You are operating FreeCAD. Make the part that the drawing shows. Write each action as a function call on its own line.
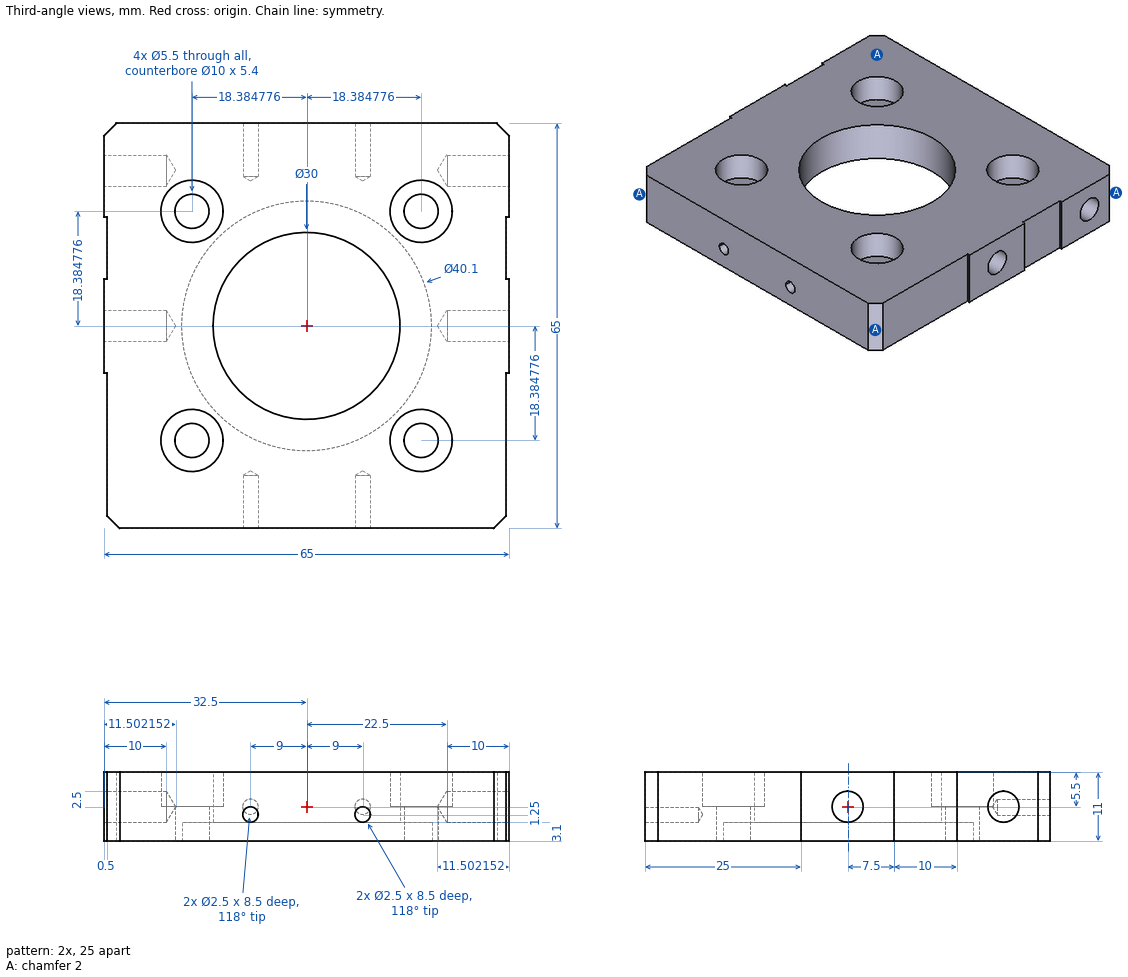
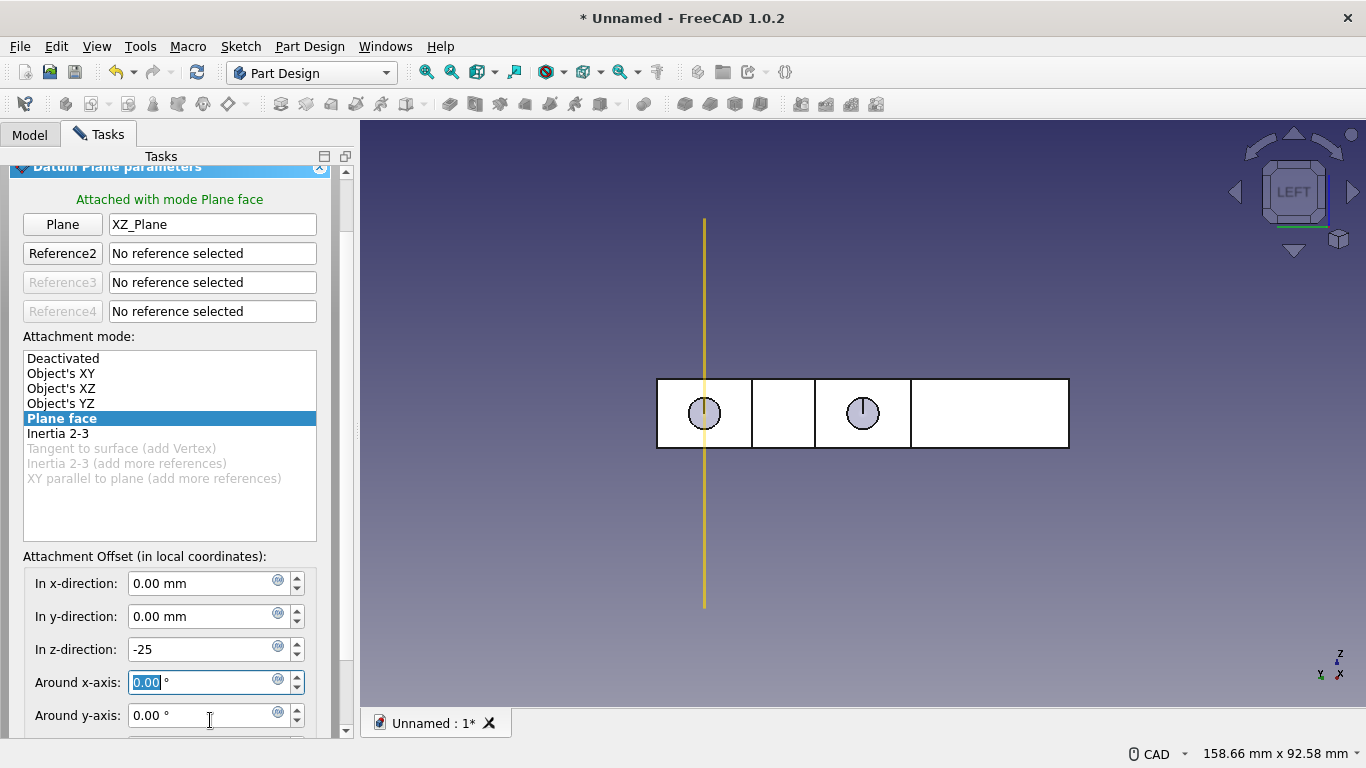
scroll(346, 452, up, 2)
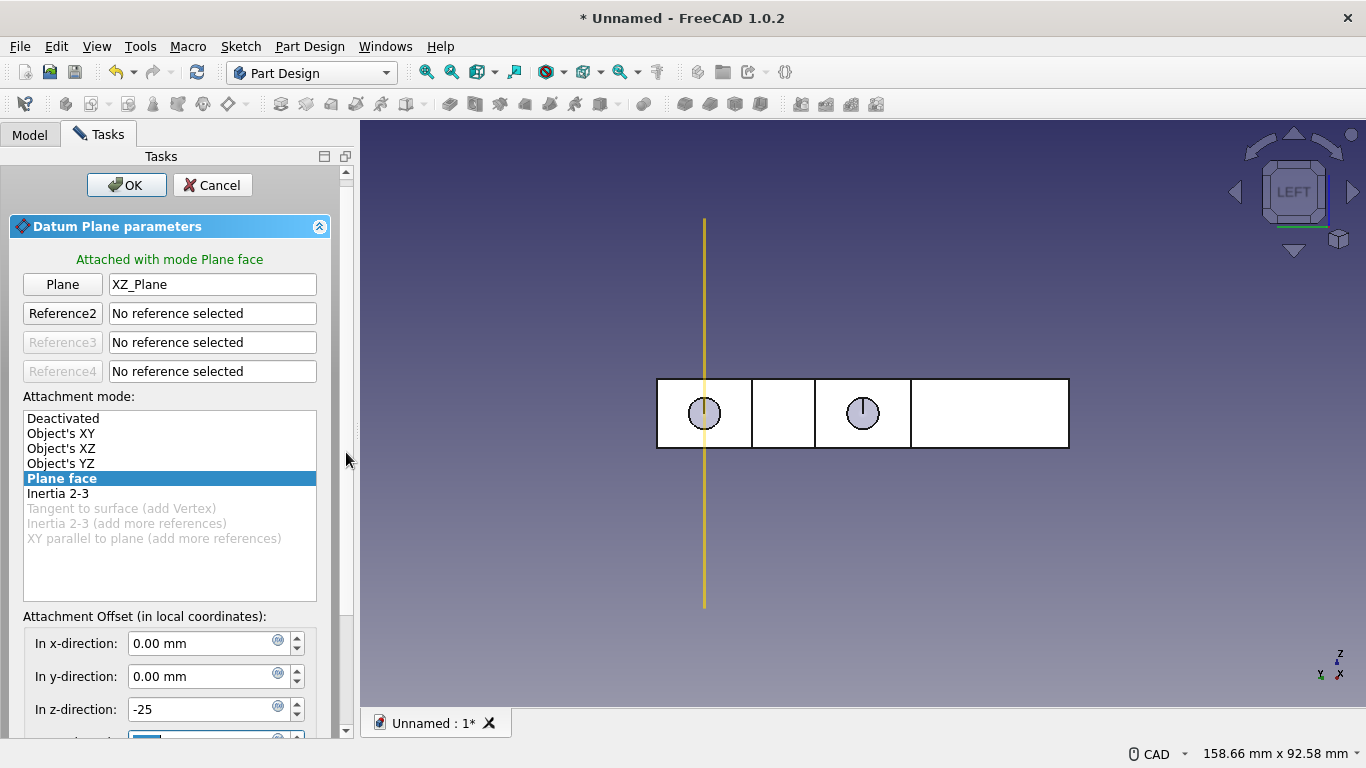
click(127, 195)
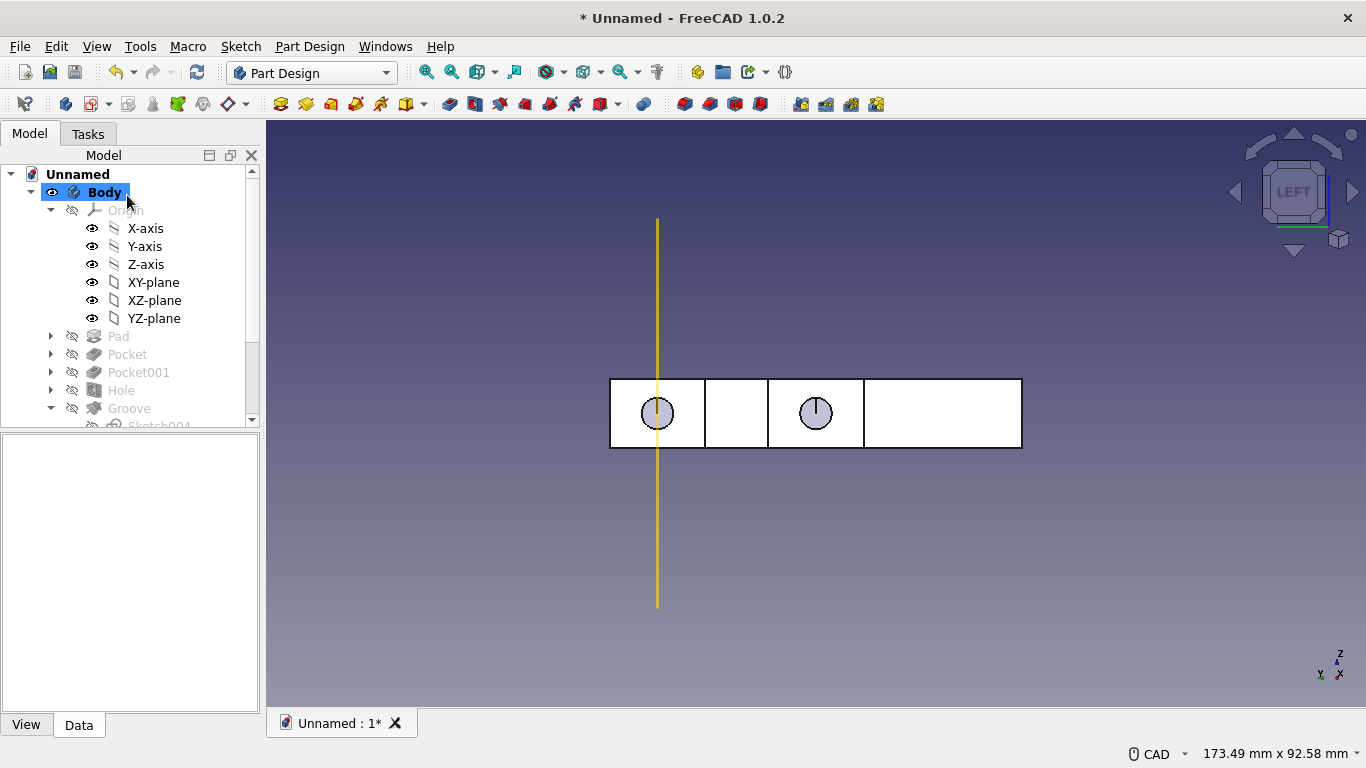
scroll(101, 296, down, 3)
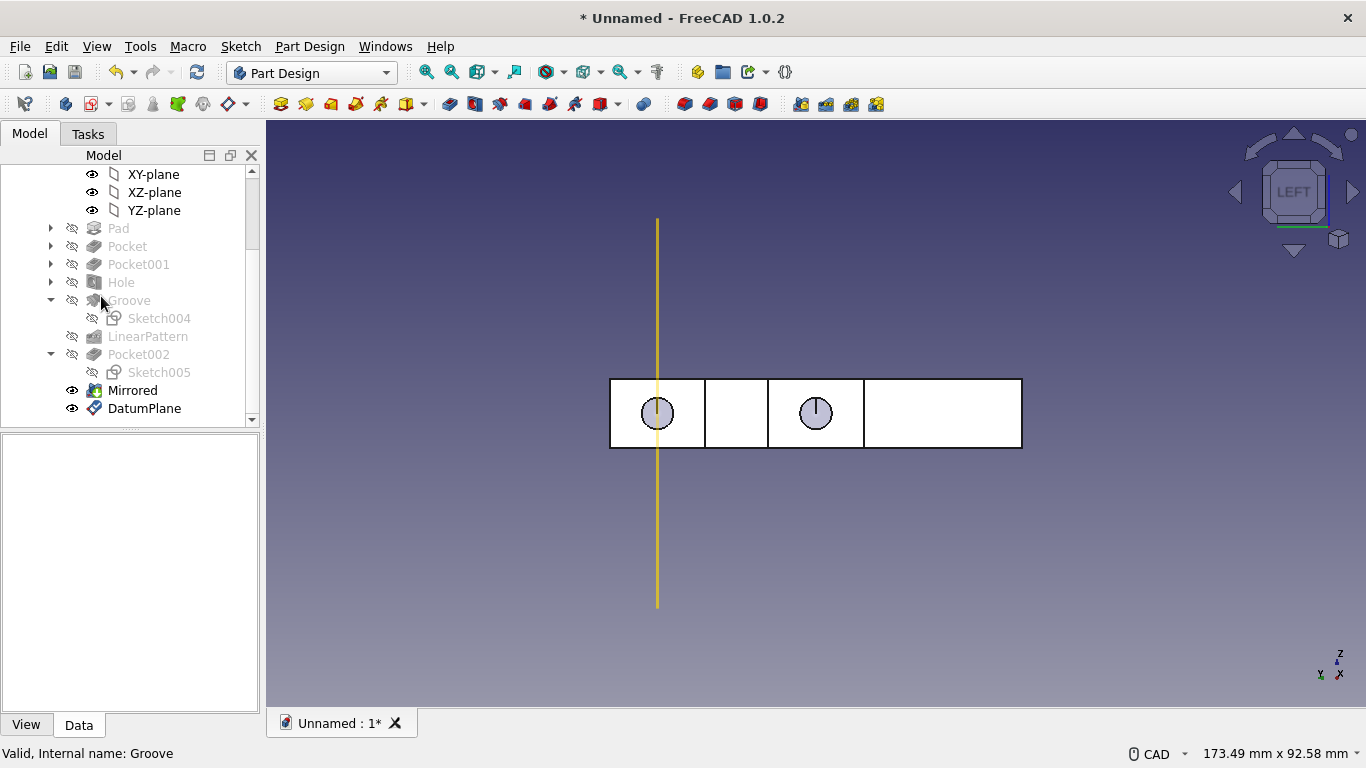
click(117, 408)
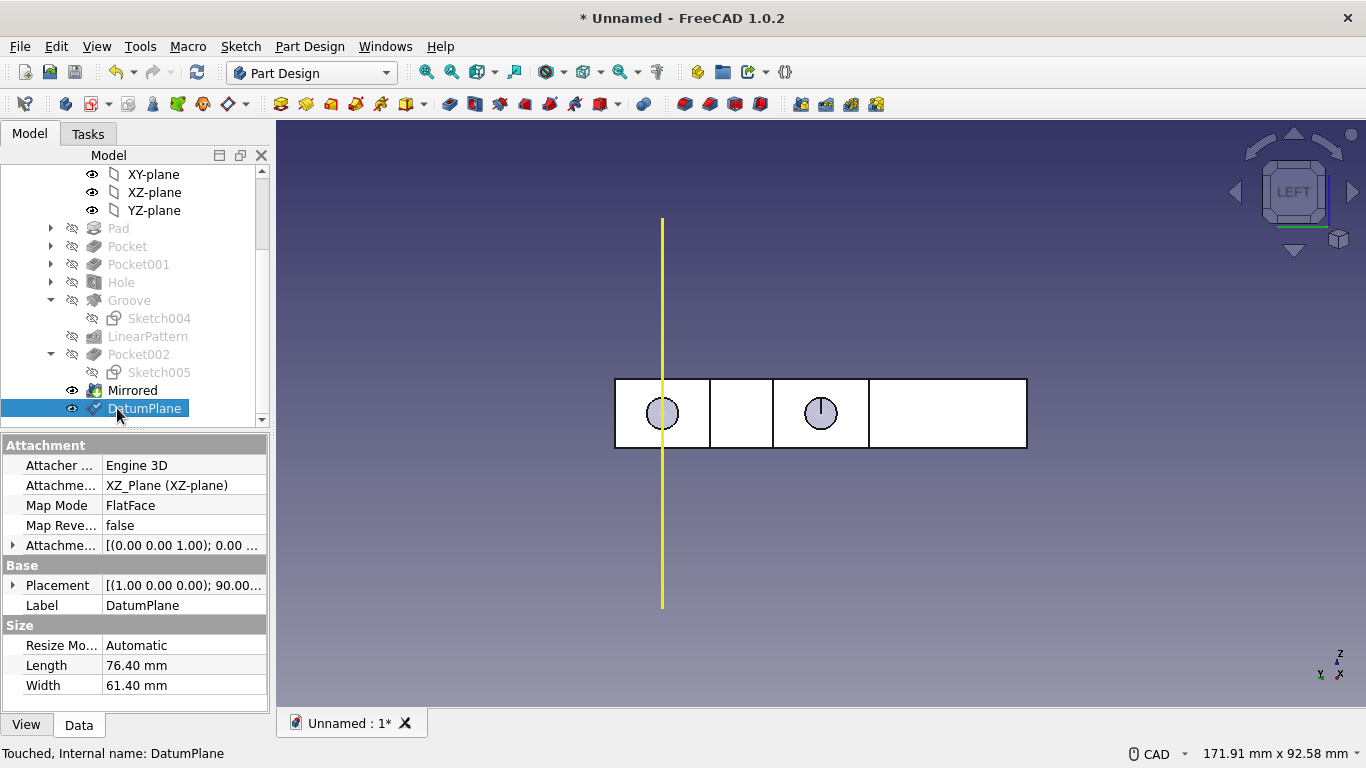
click(90, 104)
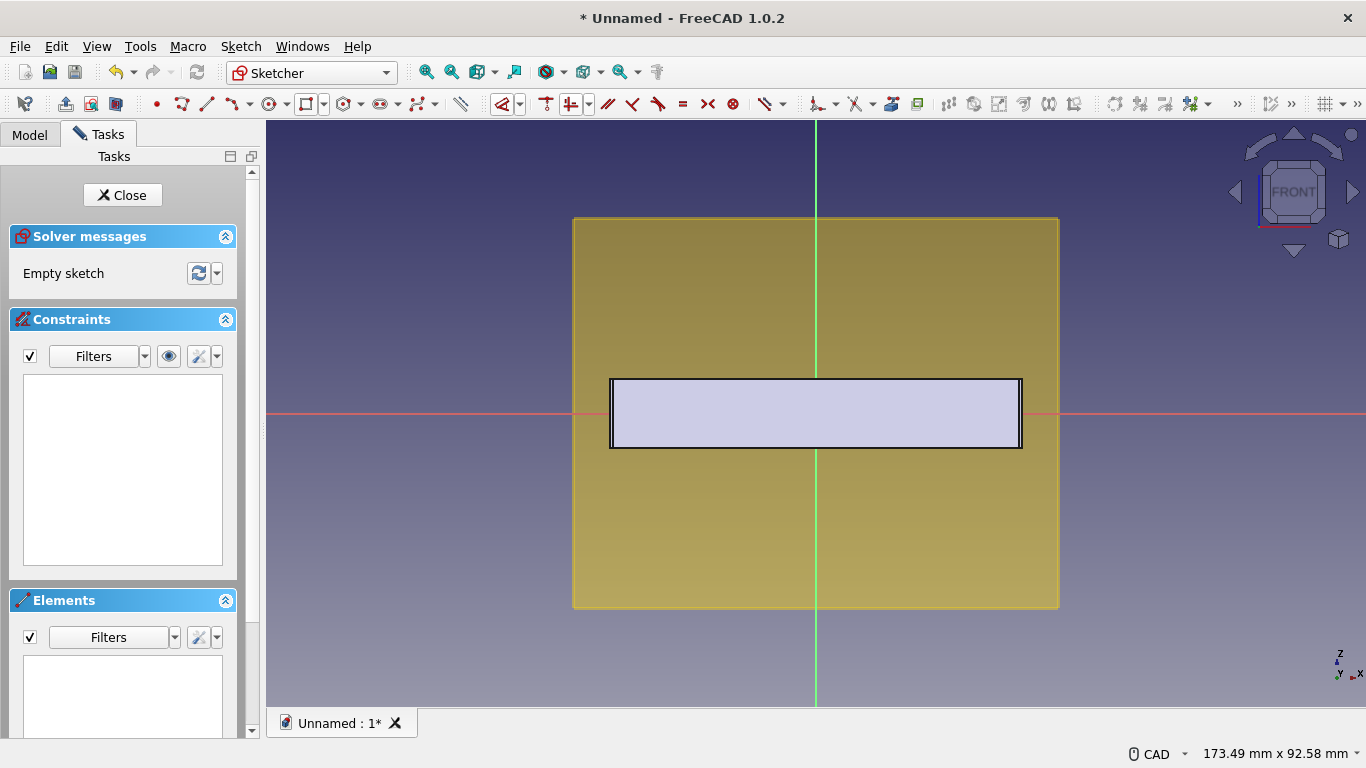
click(116, 104)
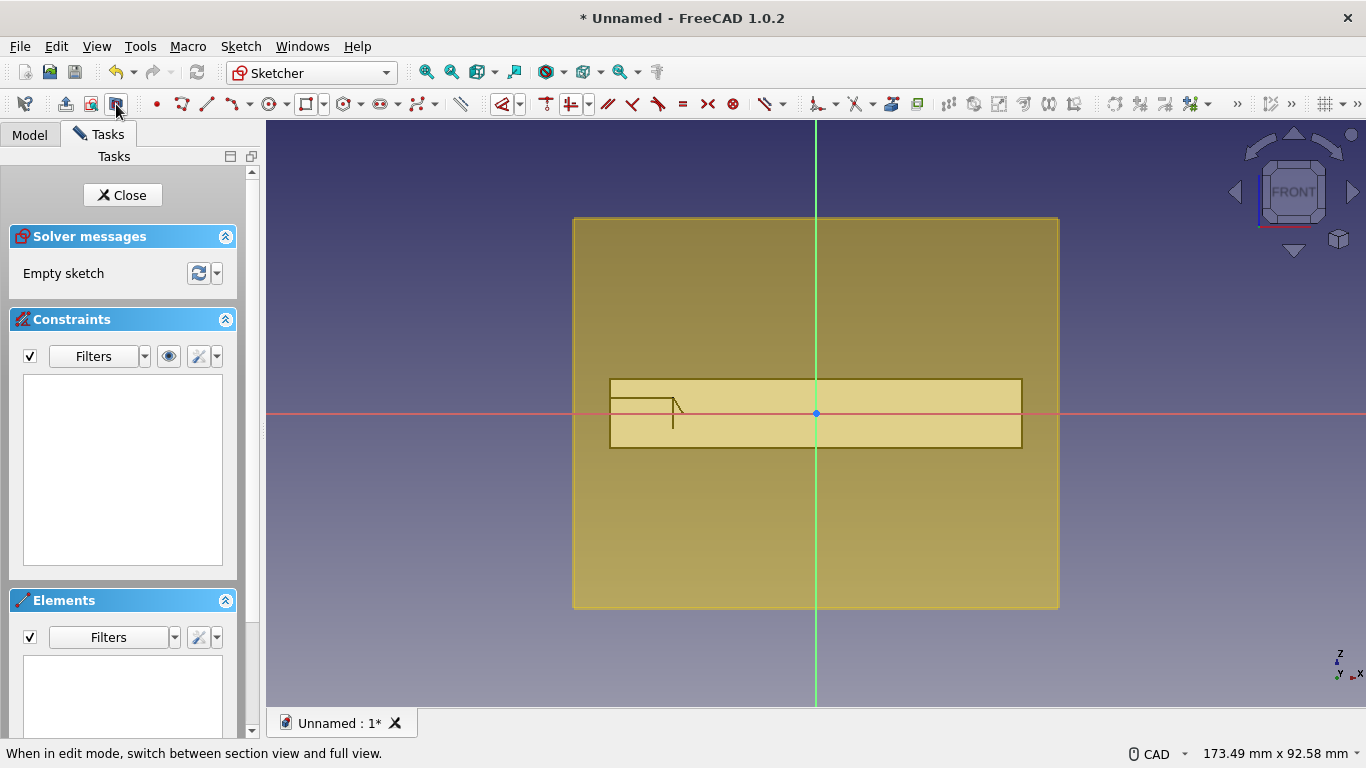
scroll(1015, 405, up, 11)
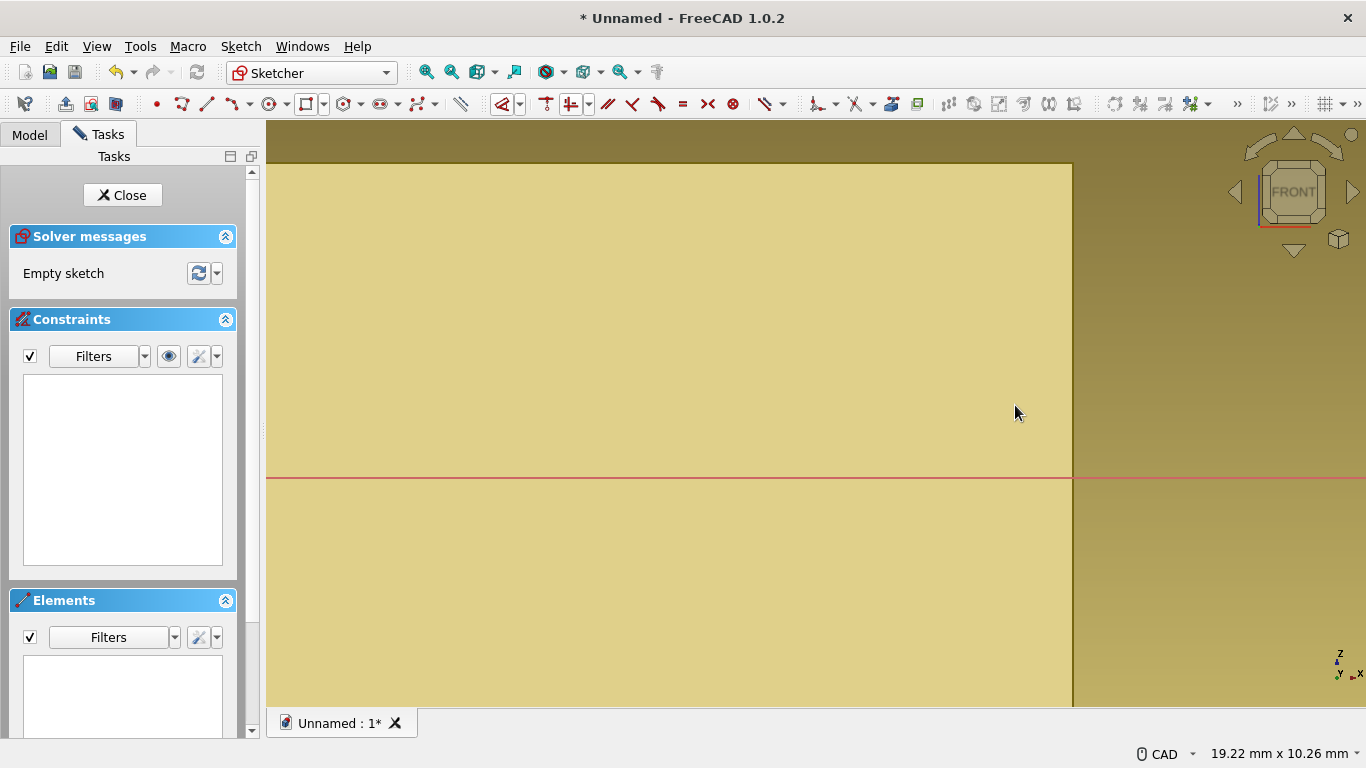
click(182, 104)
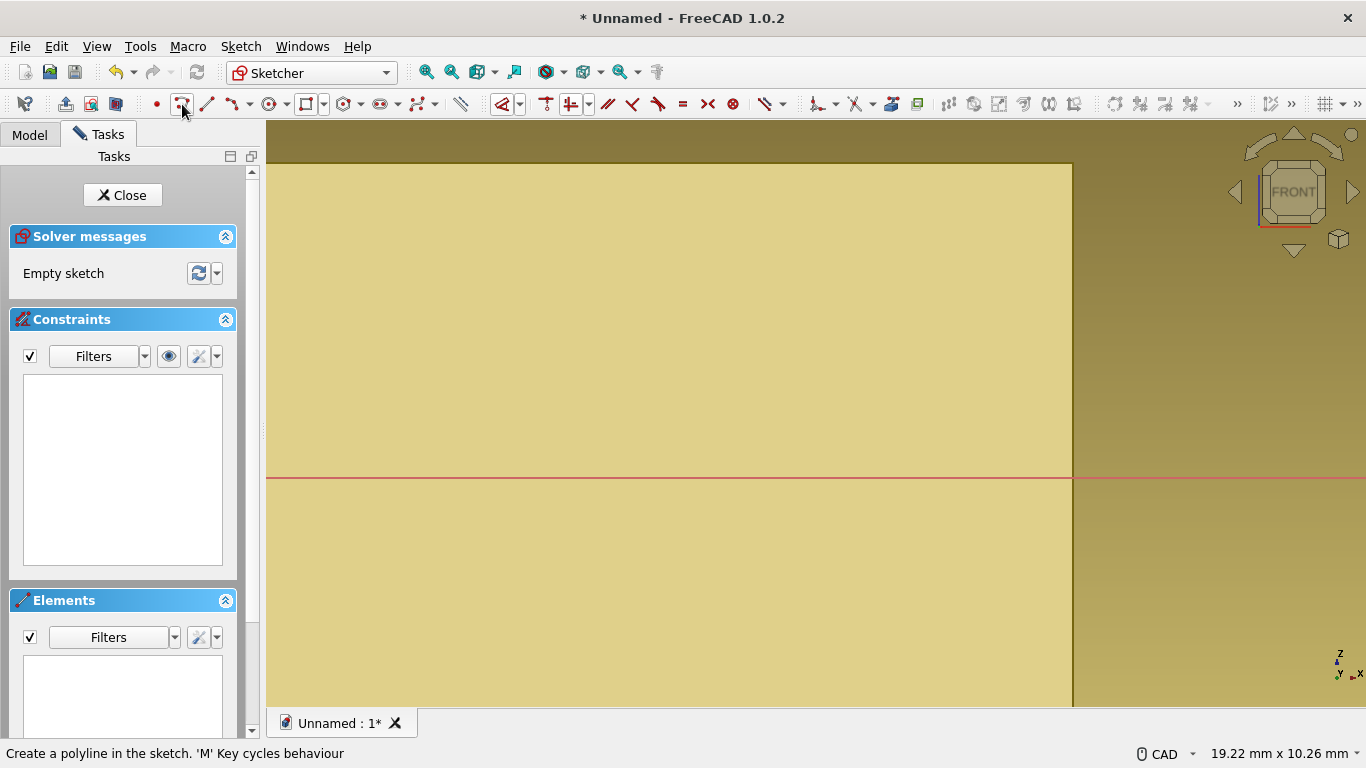
click(415, 478)
click(501, 335)
click(1073, 335)
click(1073, 469)
click(415, 478)
key(Escape)
key(Escape)